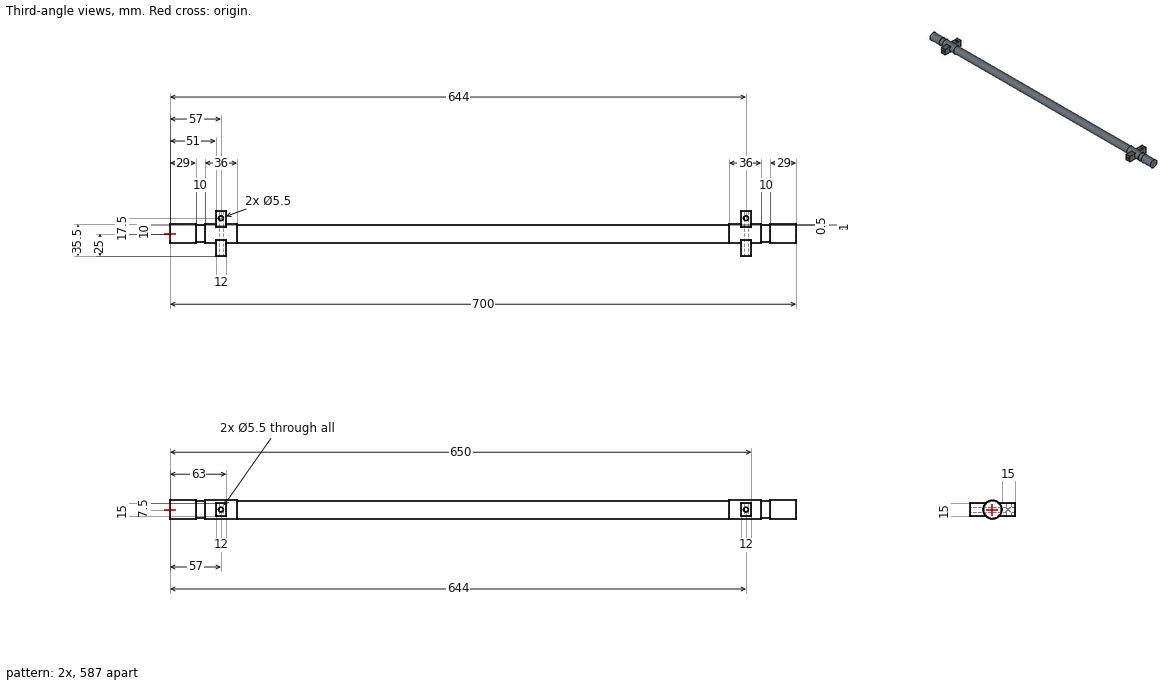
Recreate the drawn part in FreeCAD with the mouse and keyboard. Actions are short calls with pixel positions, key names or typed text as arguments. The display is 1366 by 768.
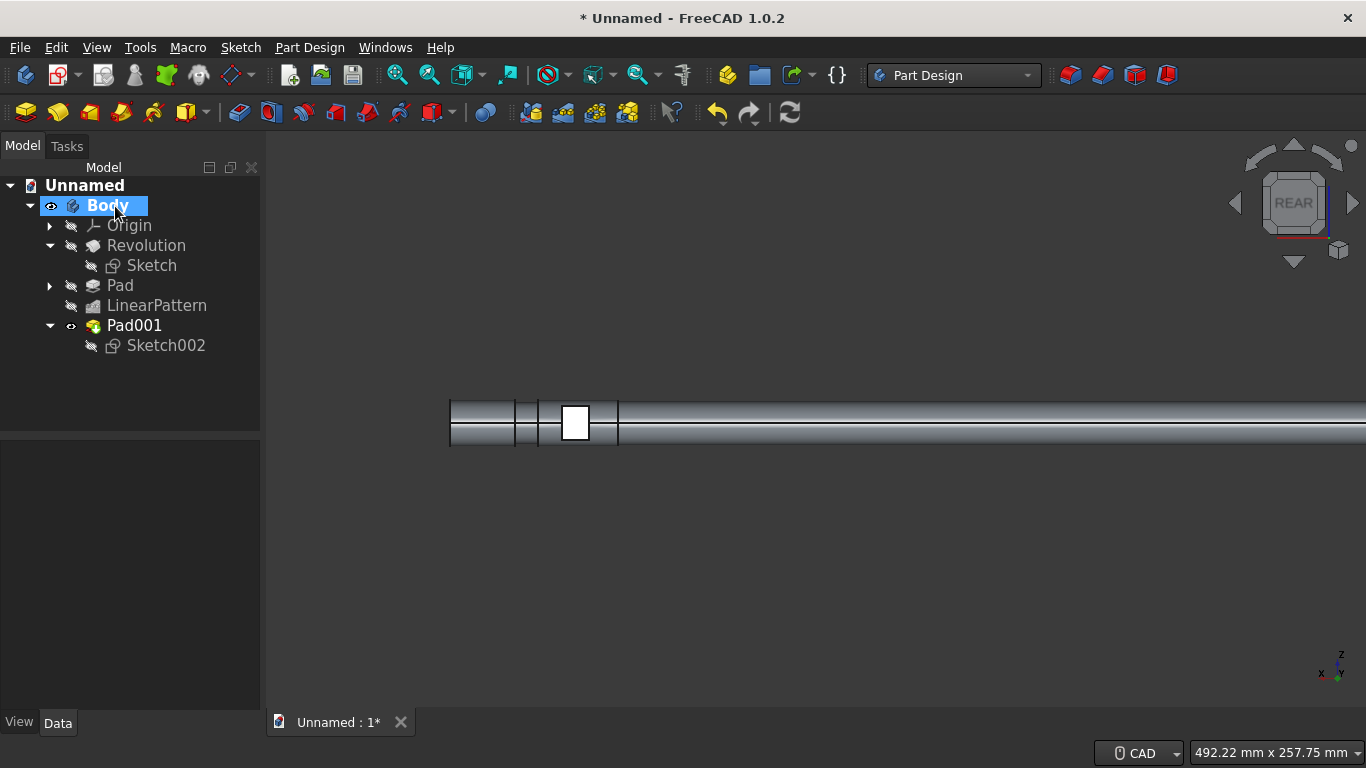
click(398, 76)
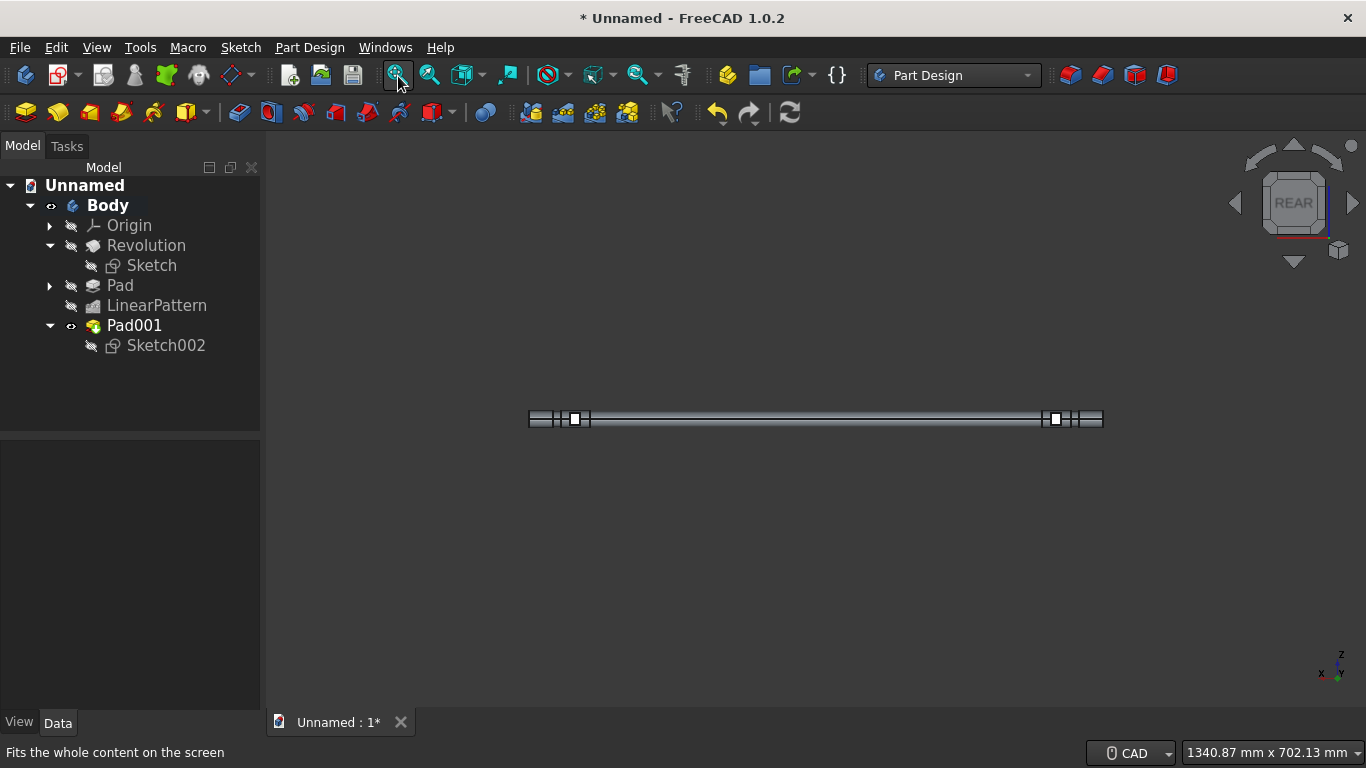
scroll(575, 418, up, 5)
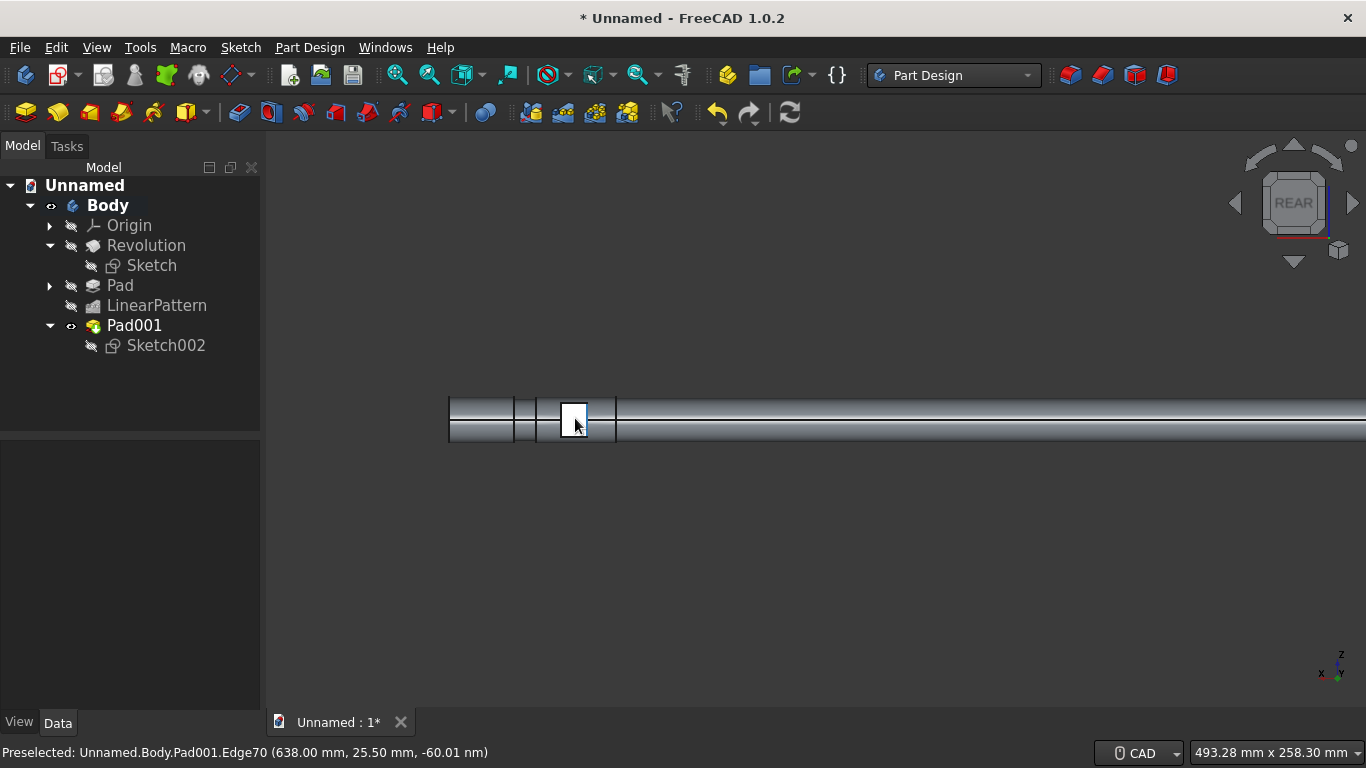
click(574, 419)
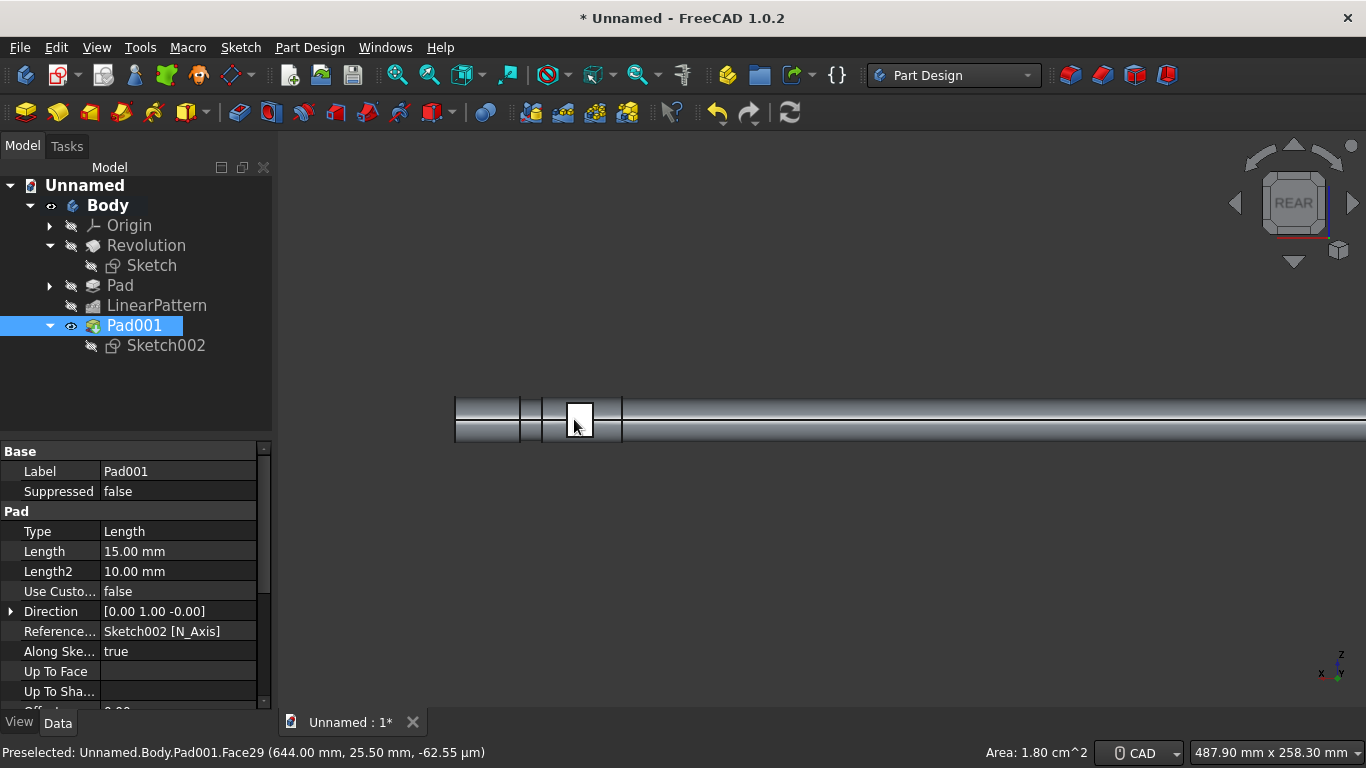
click(58, 76)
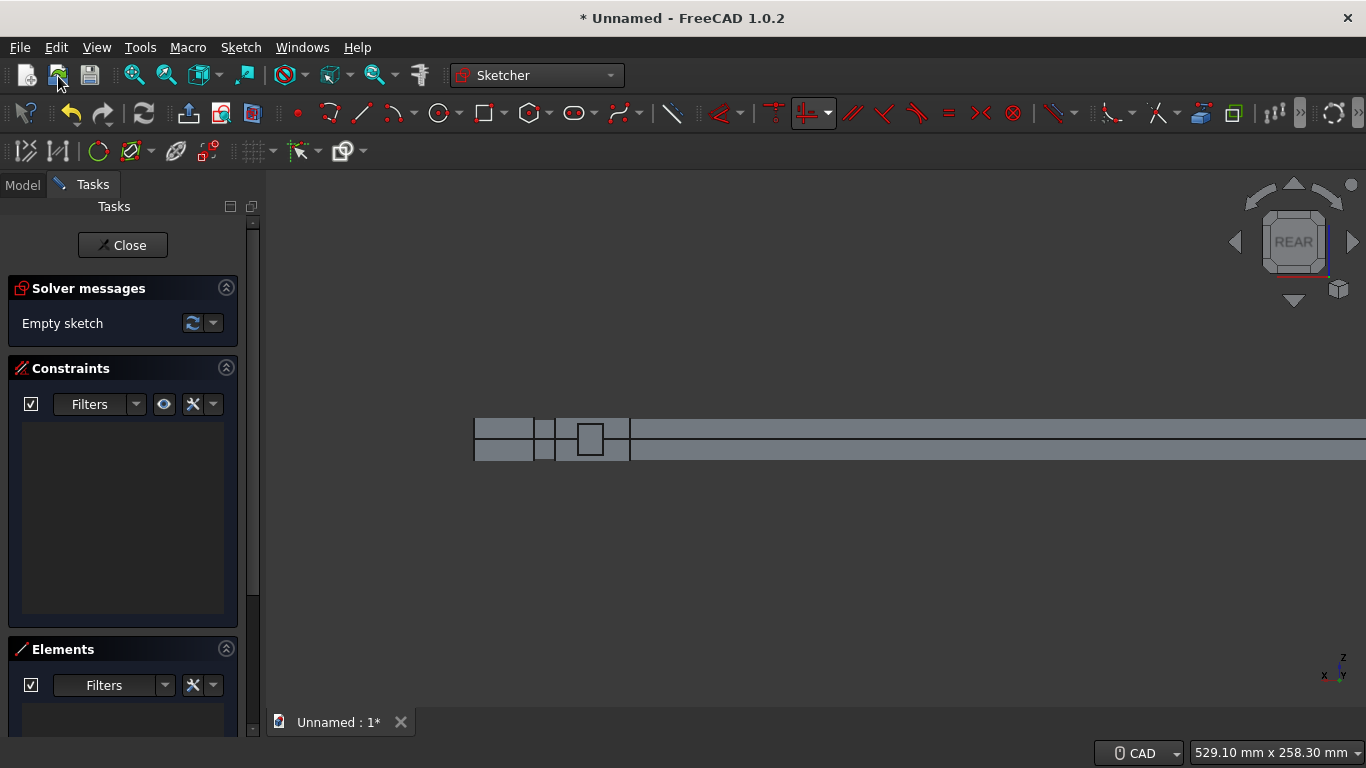
scroll(332, 438, down, 4)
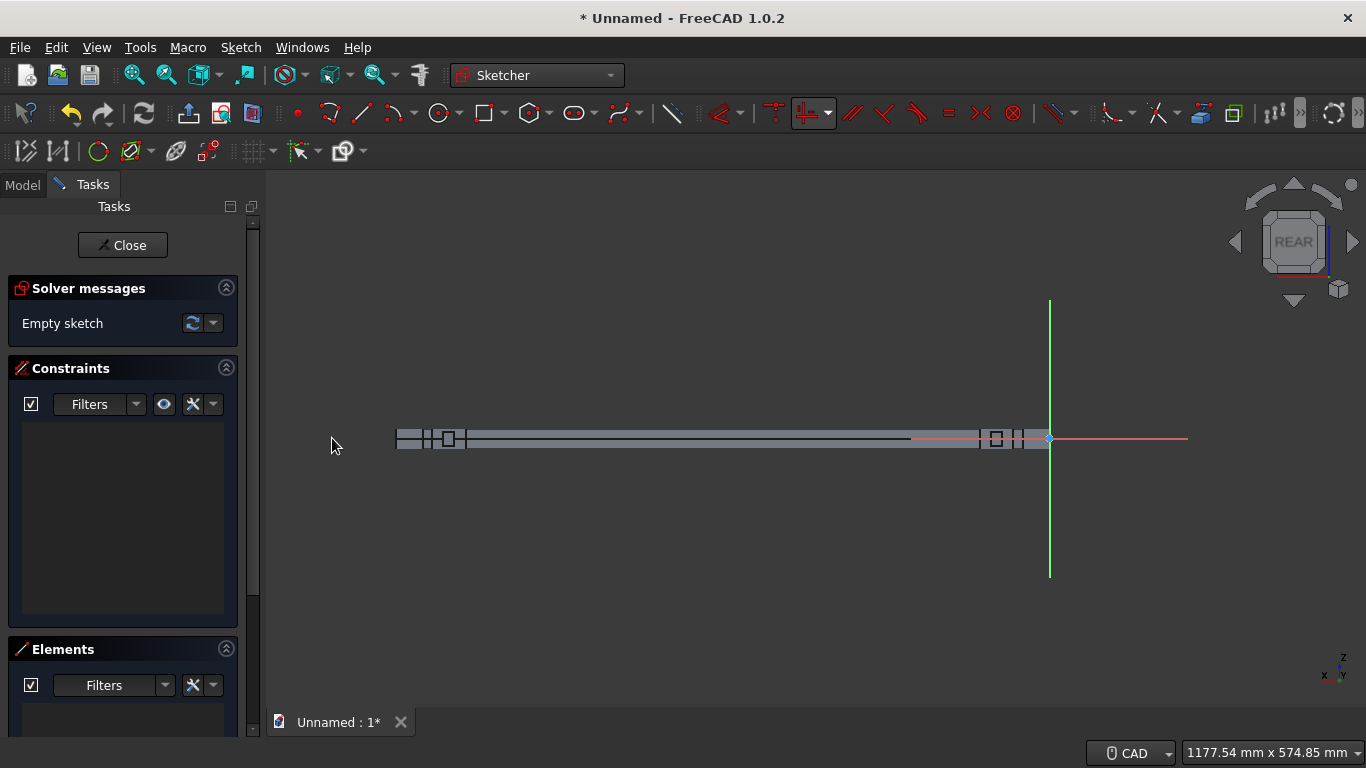
click(440, 114)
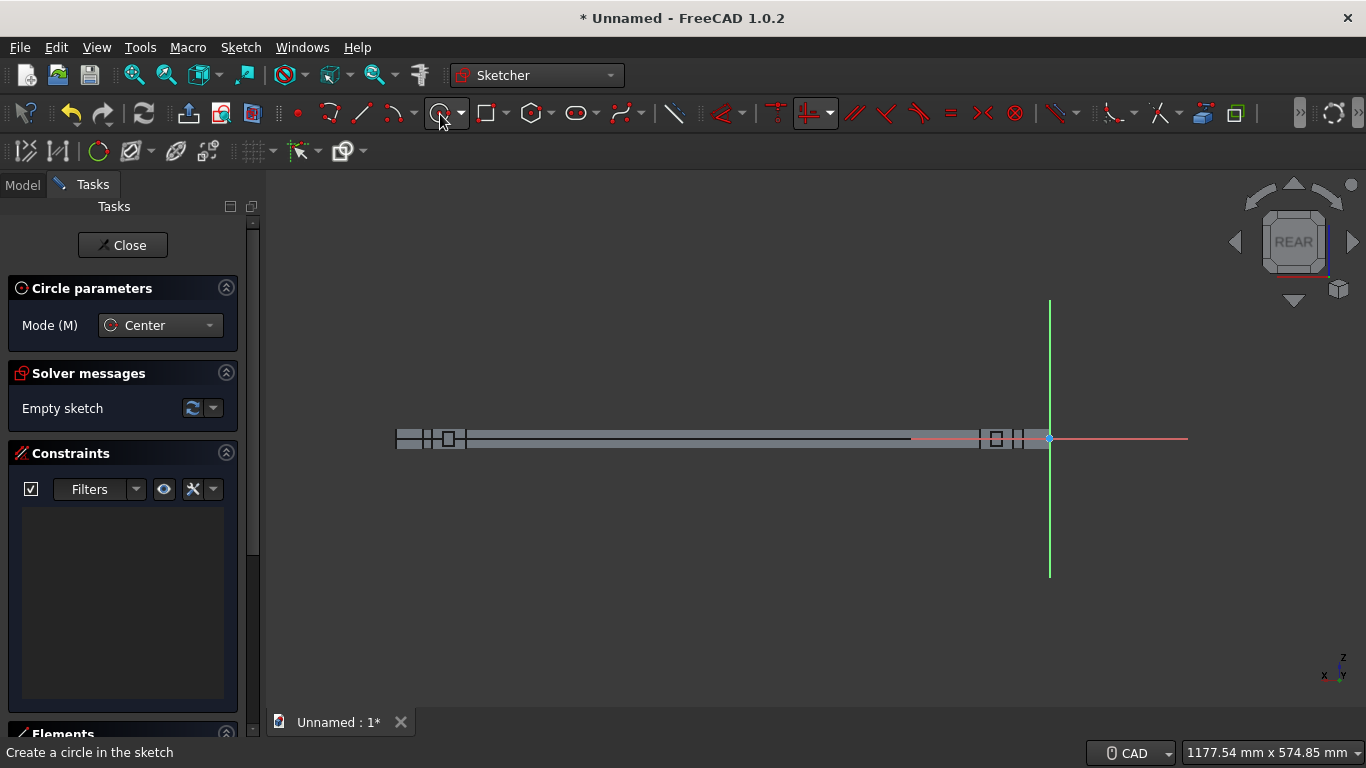
scroll(996, 439, up, 11)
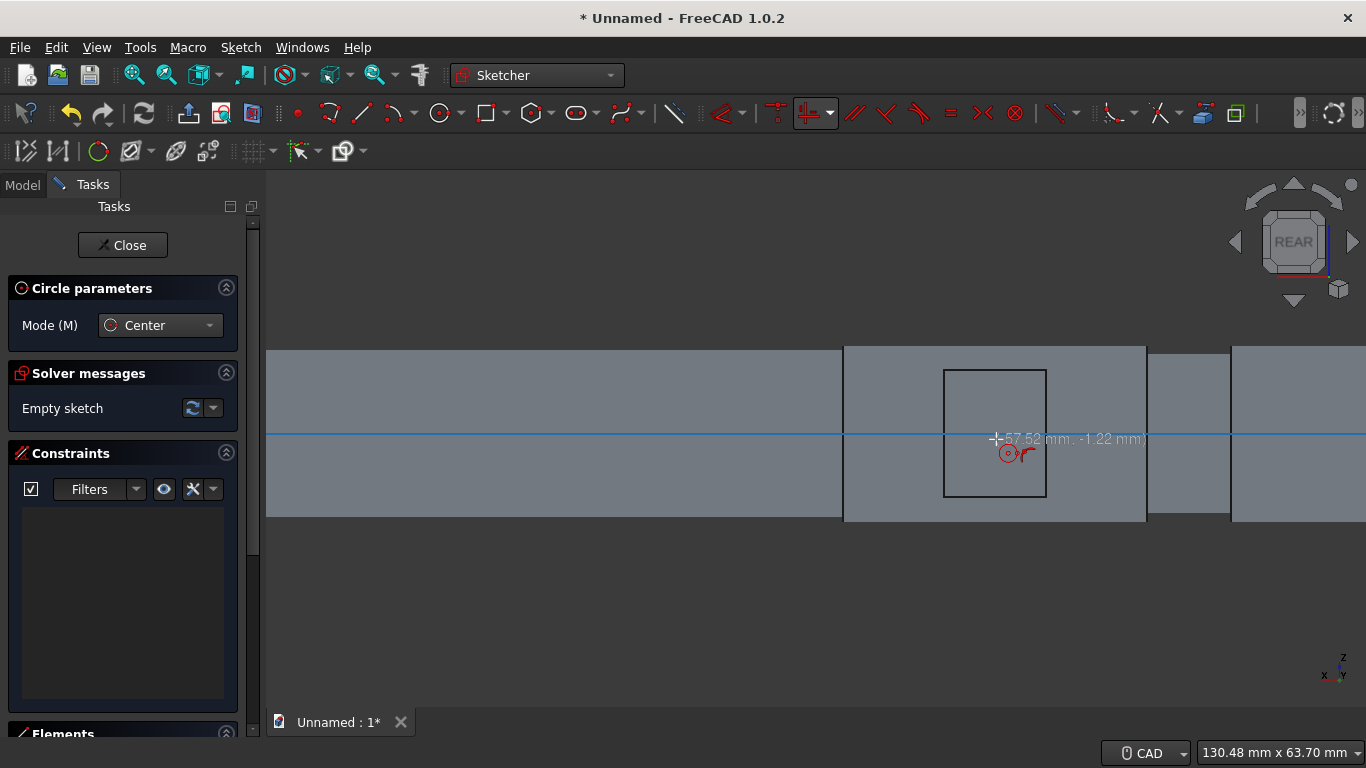
scroll(996, 439, down, 11)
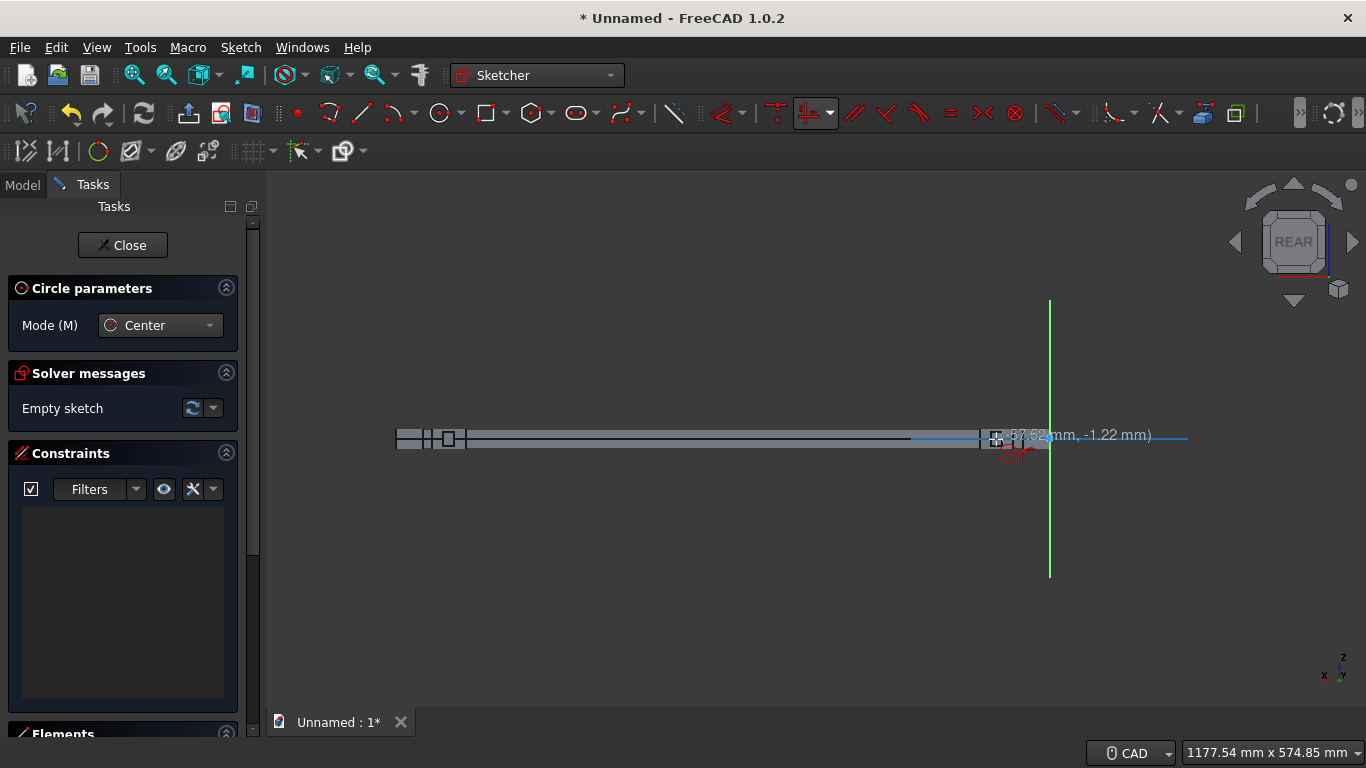
click(996, 439)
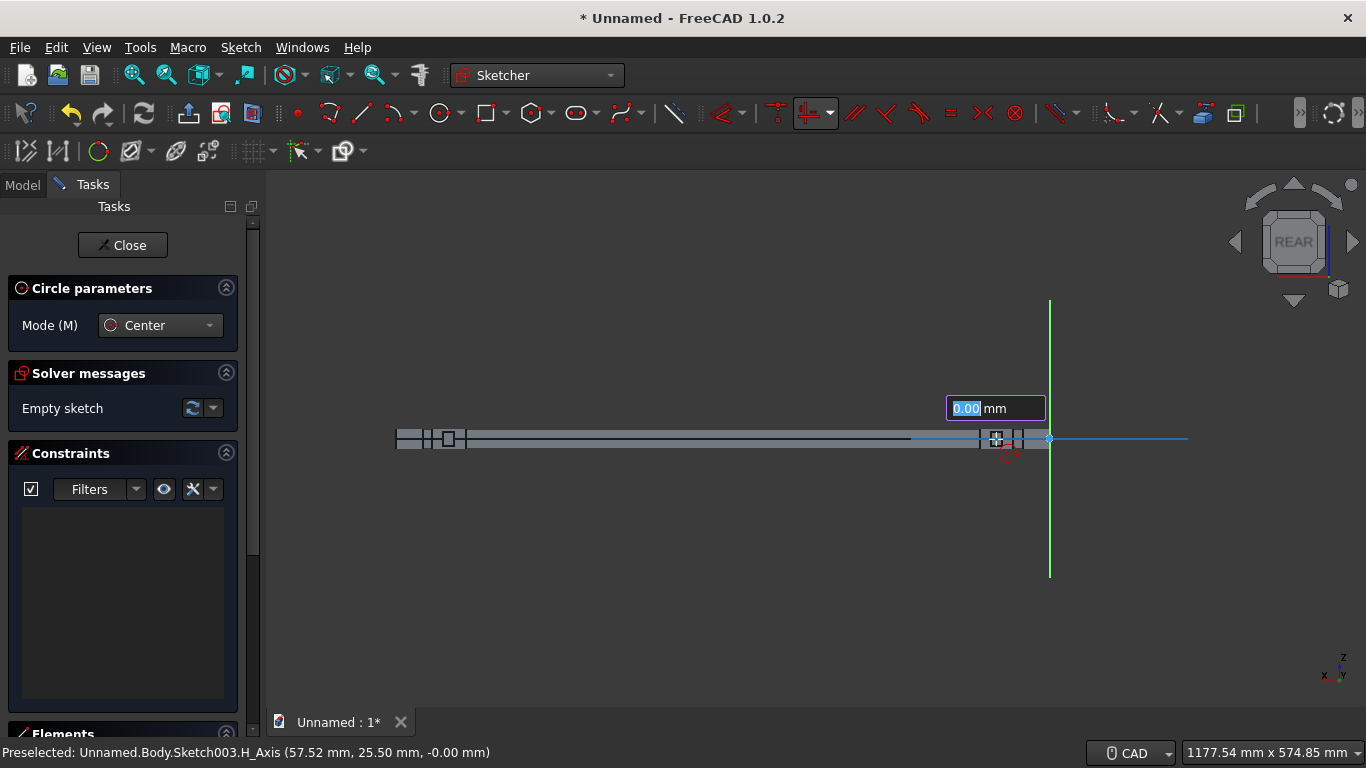
scroll(997, 436, up, 10)